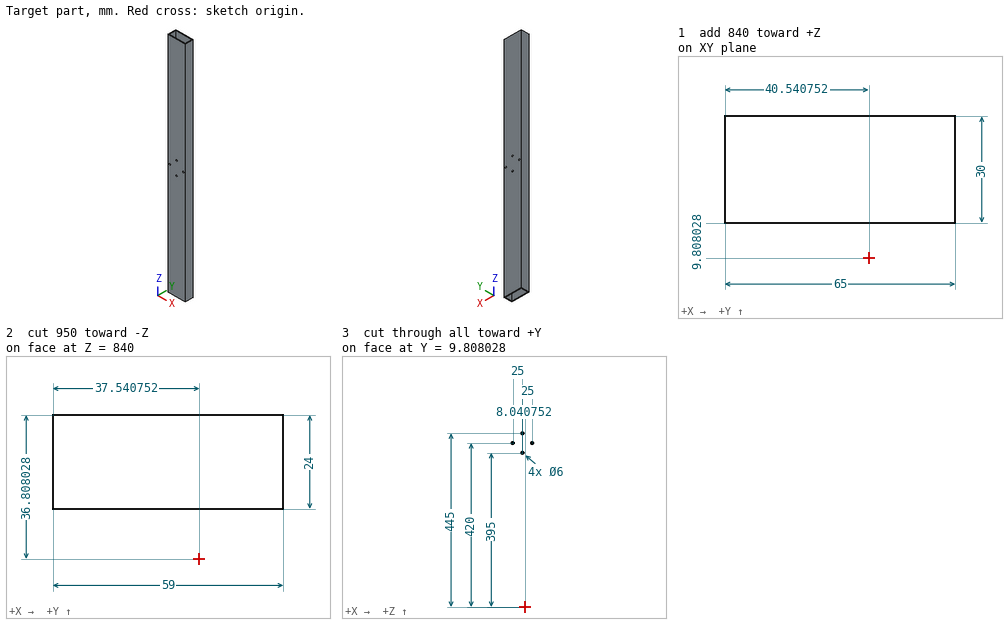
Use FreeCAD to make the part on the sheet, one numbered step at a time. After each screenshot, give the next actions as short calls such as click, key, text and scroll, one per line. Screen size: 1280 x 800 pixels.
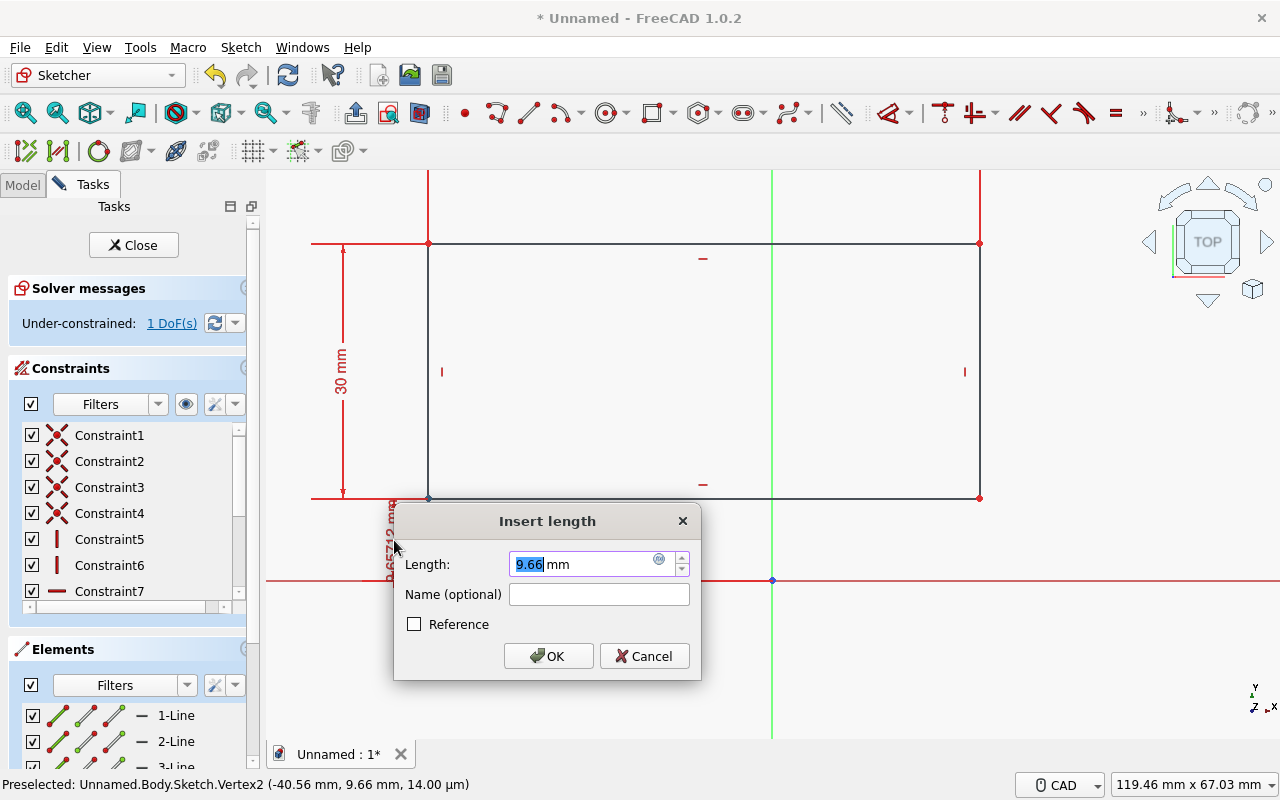
text(9.808028)
key(Return)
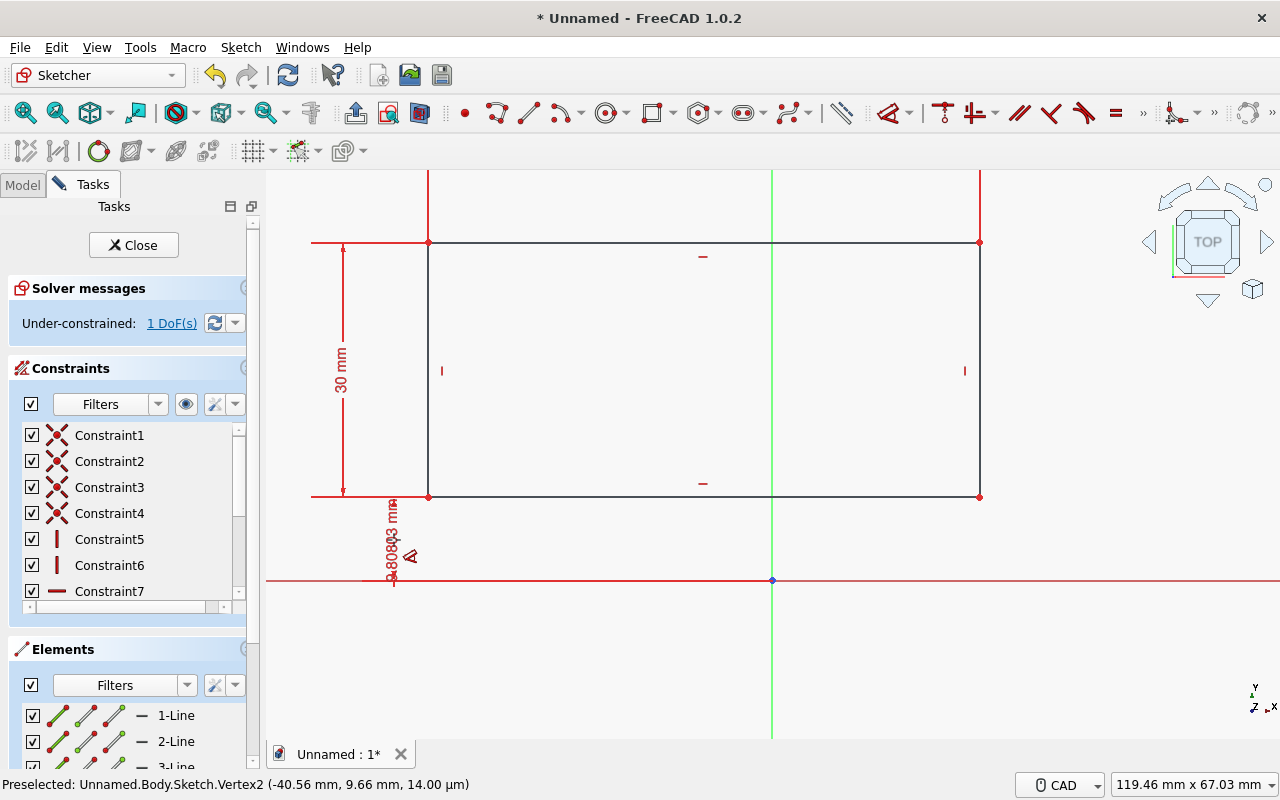
click(428, 243)
click(600, 209)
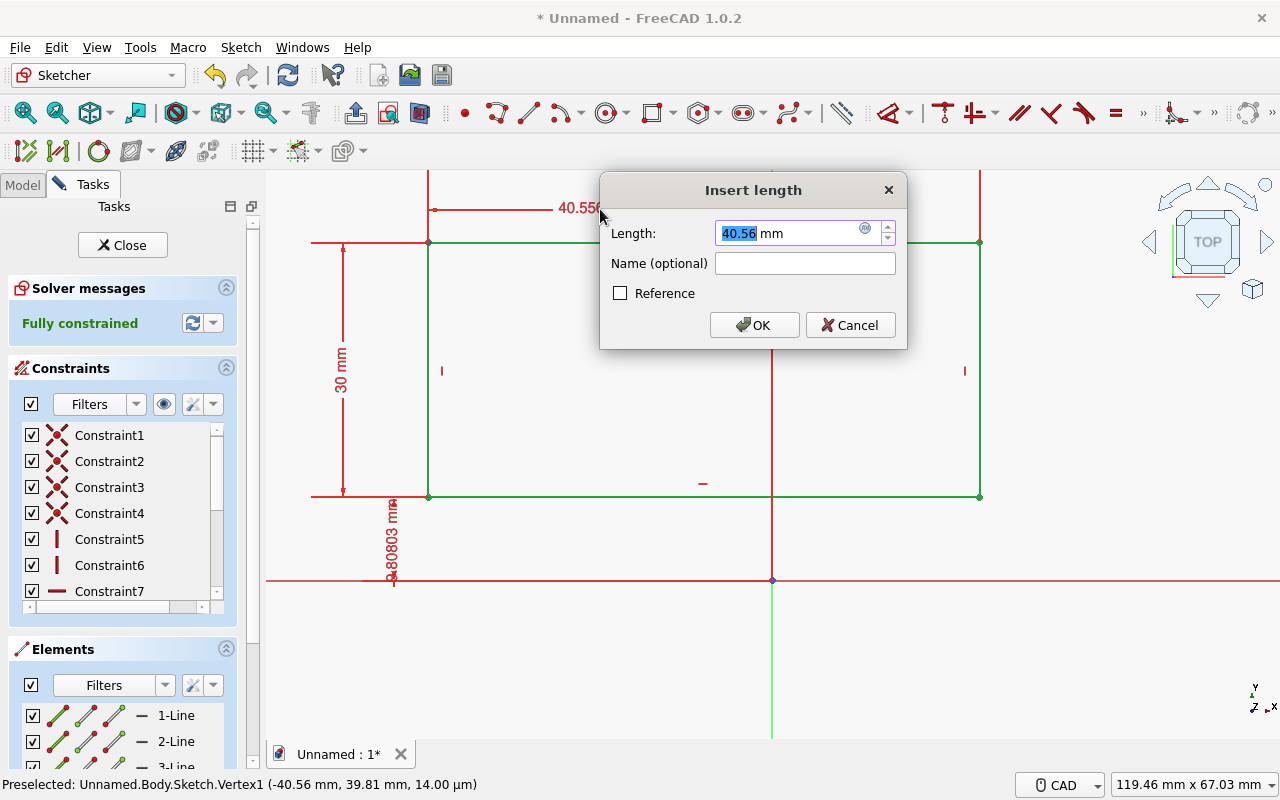
text(40.540752)
key(Return)
key(Escape)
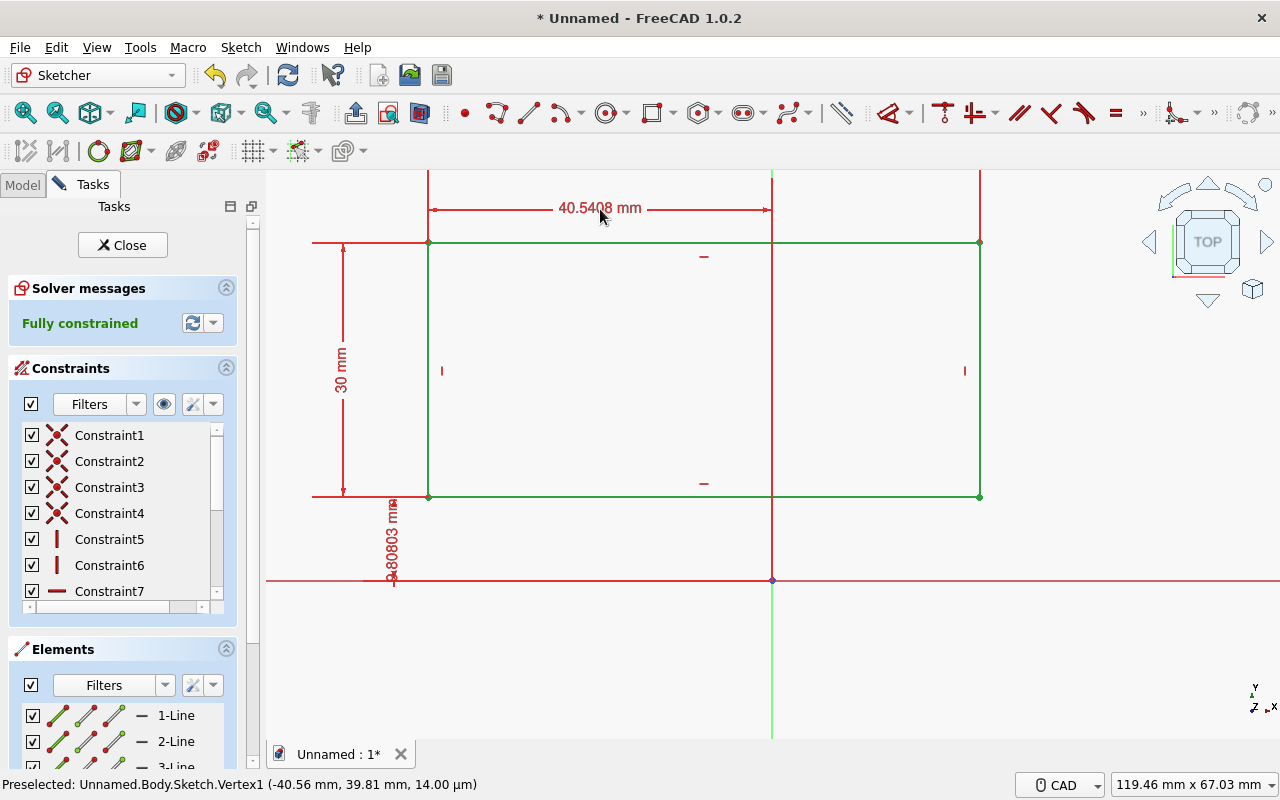
click(123, 245)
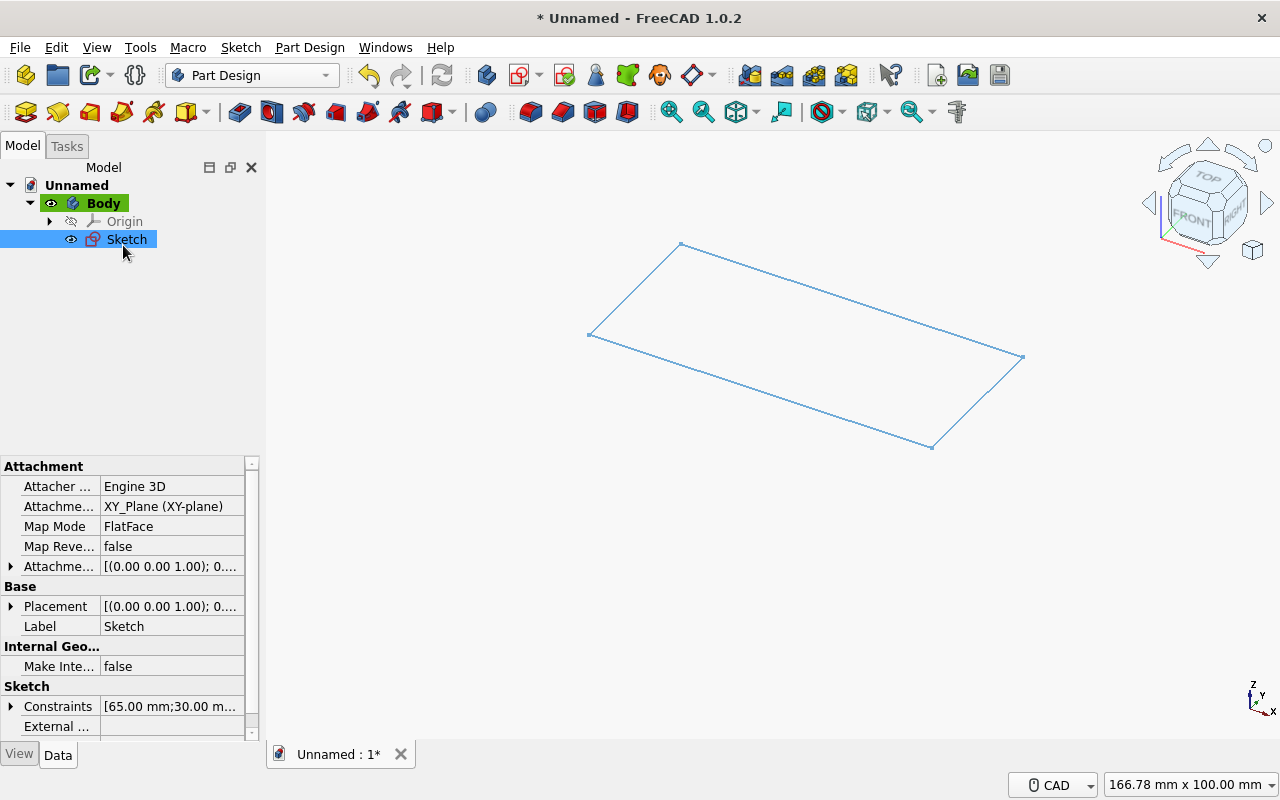
click(26, 112)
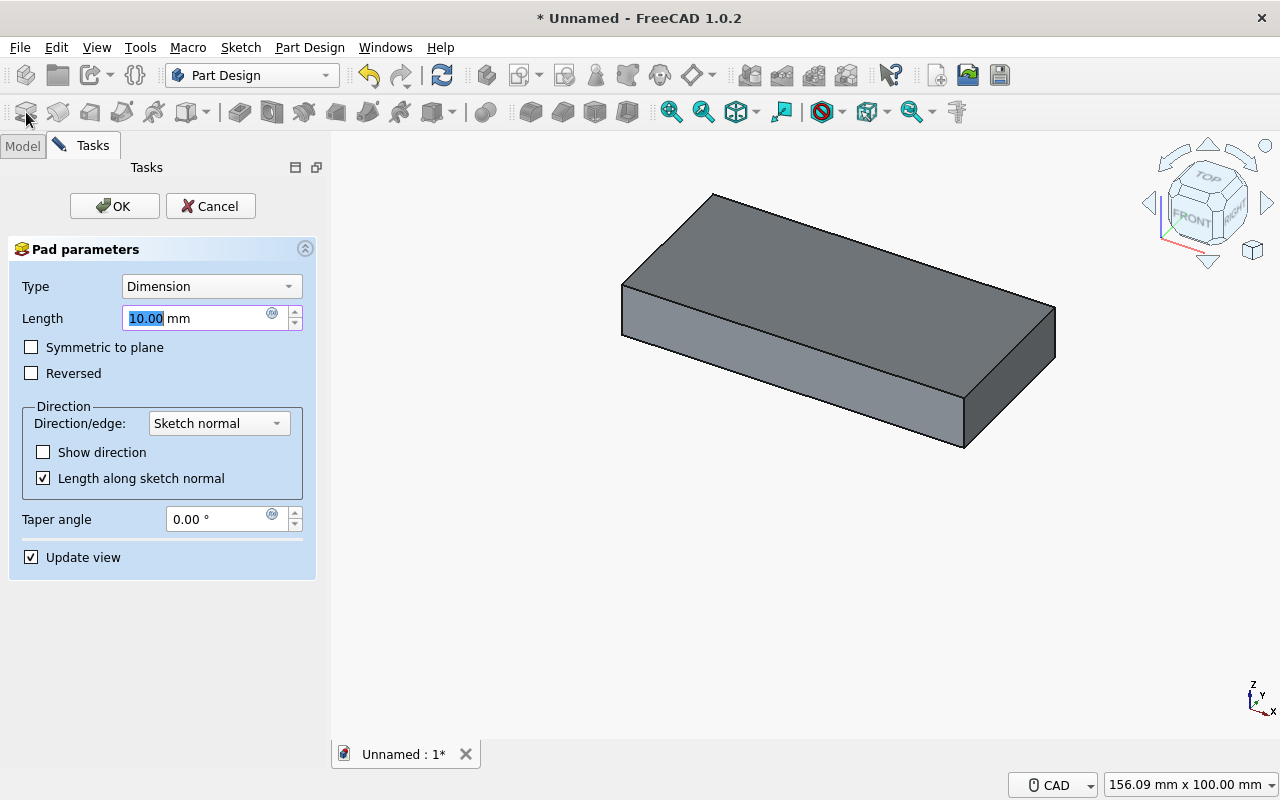
text(840)
key(Tab)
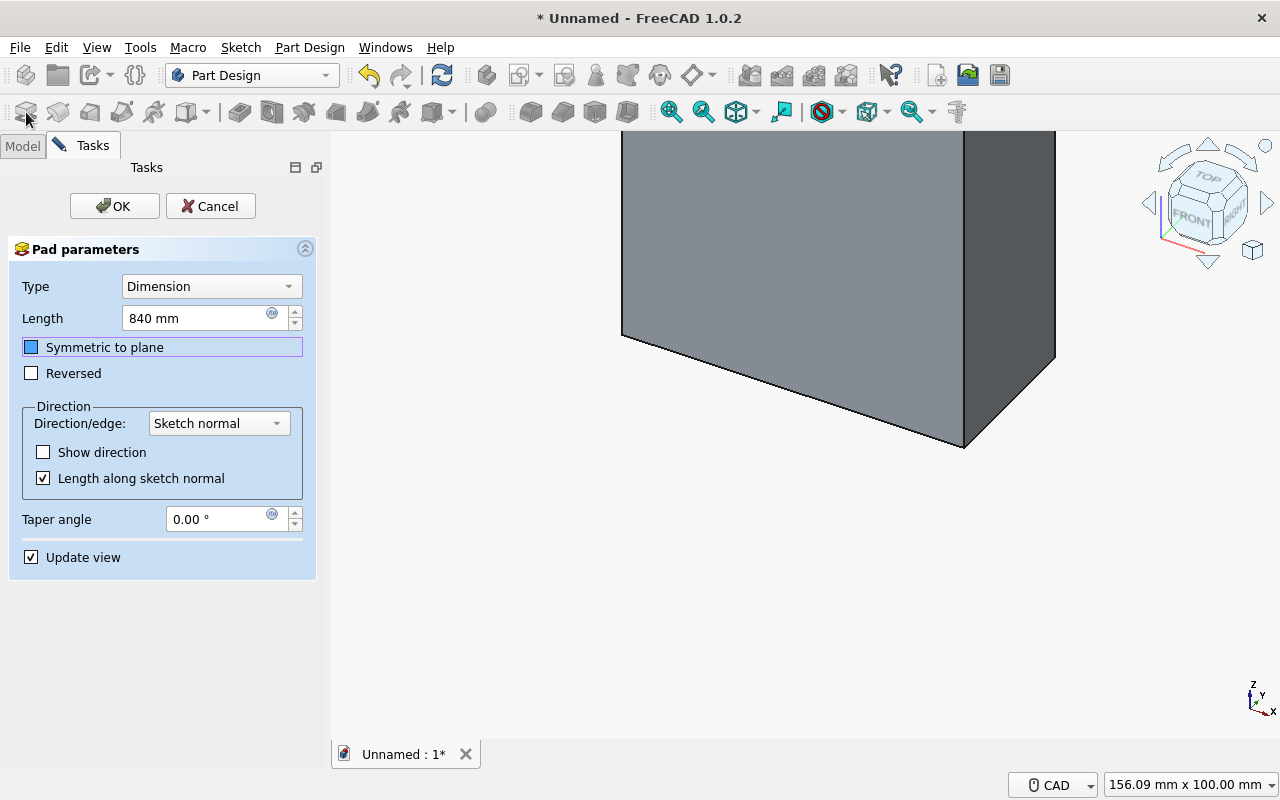
click(115, 206)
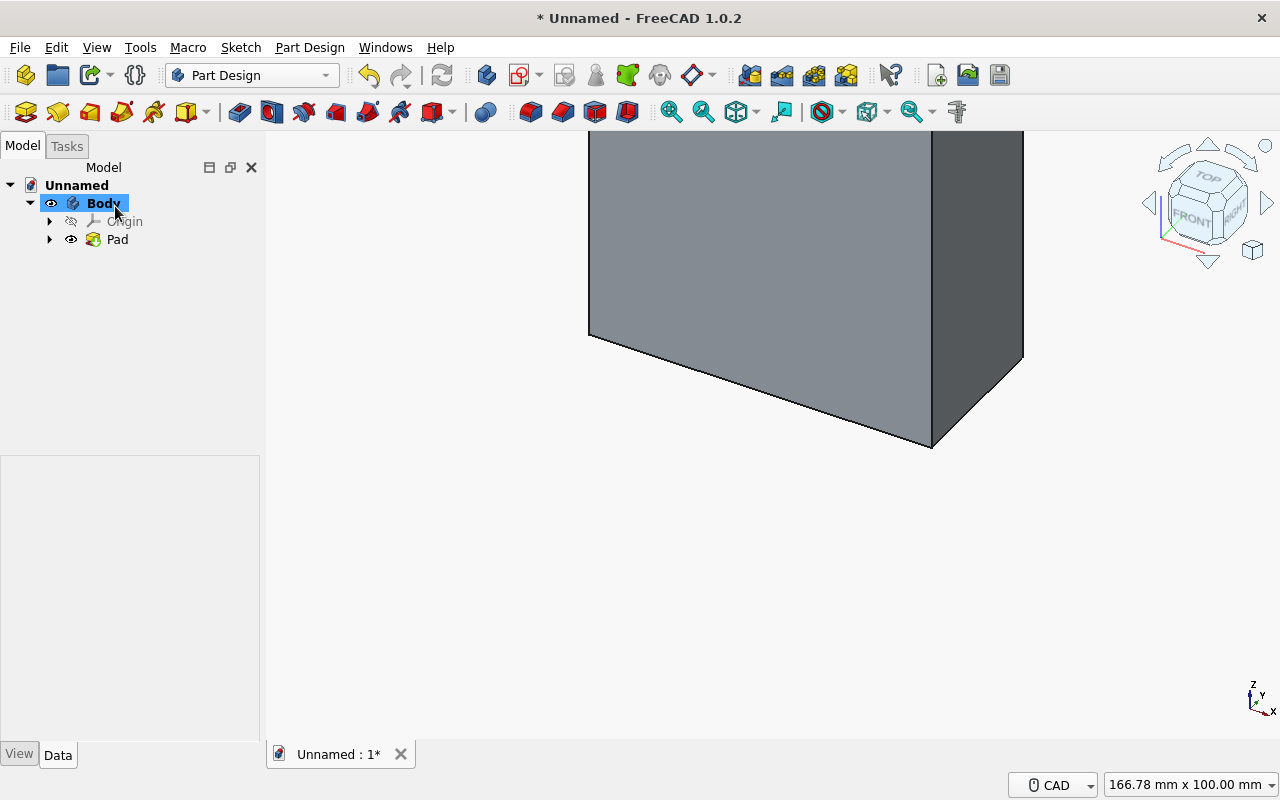
click(672, 112)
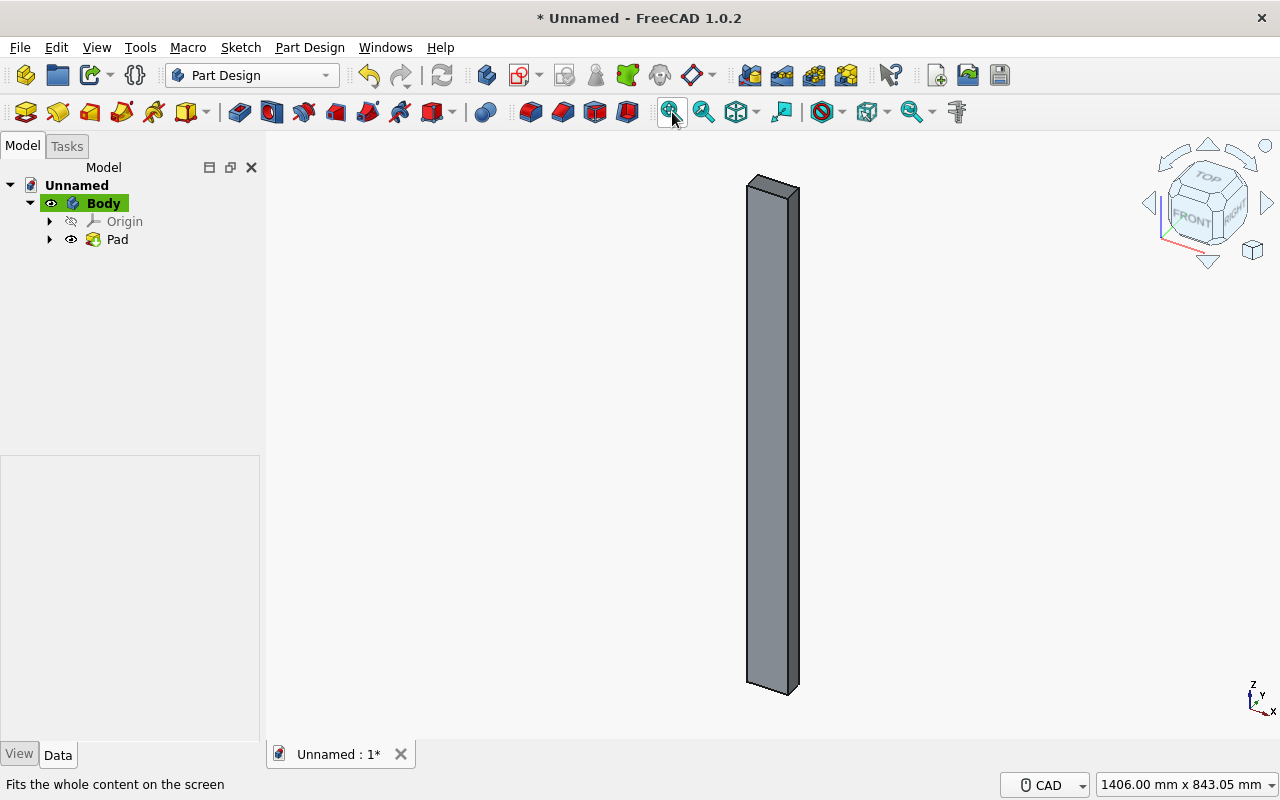
click(780, 186)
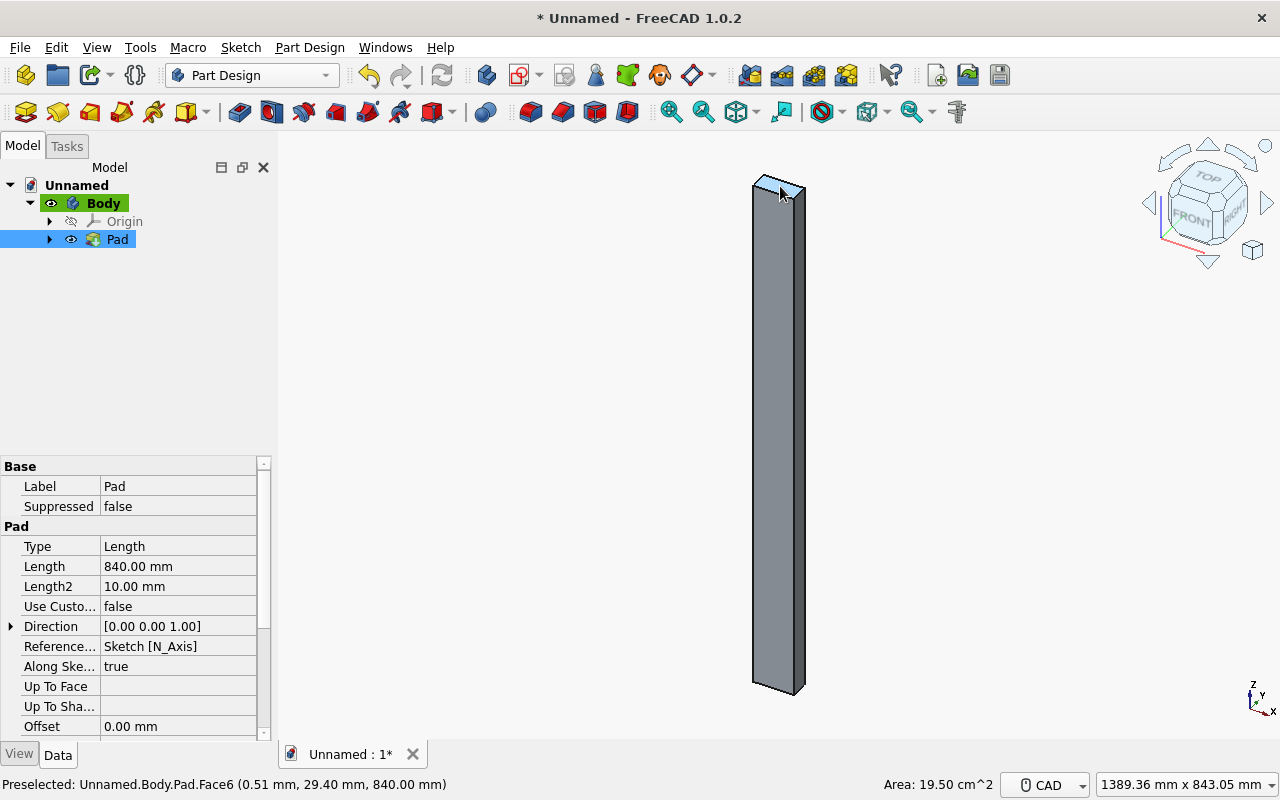
click(520, 76)